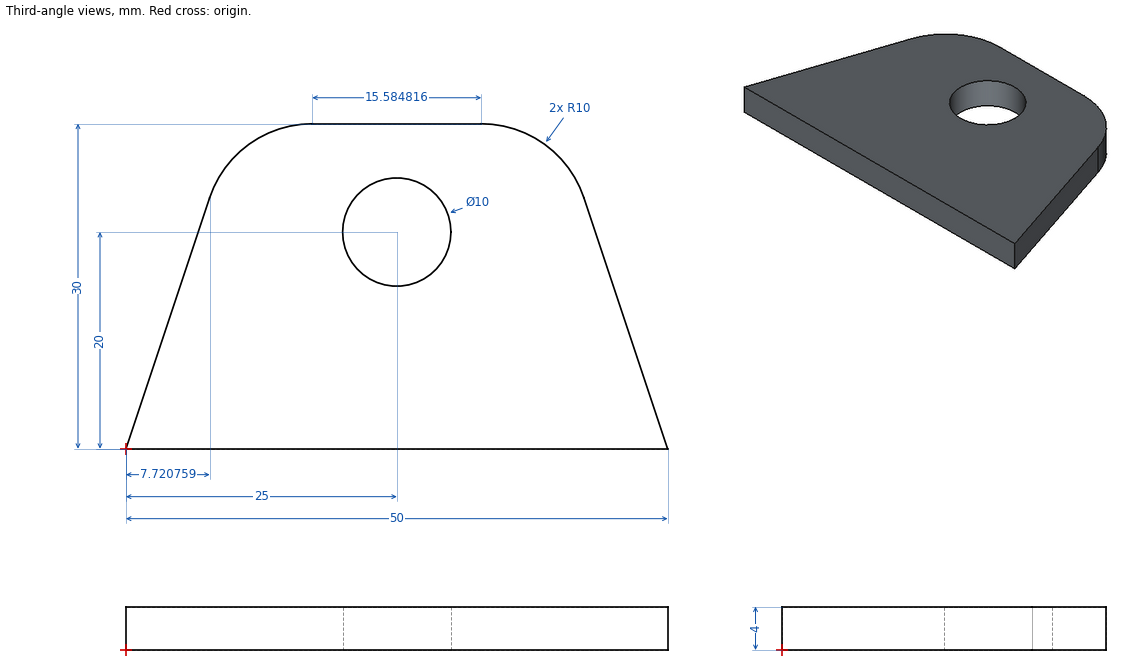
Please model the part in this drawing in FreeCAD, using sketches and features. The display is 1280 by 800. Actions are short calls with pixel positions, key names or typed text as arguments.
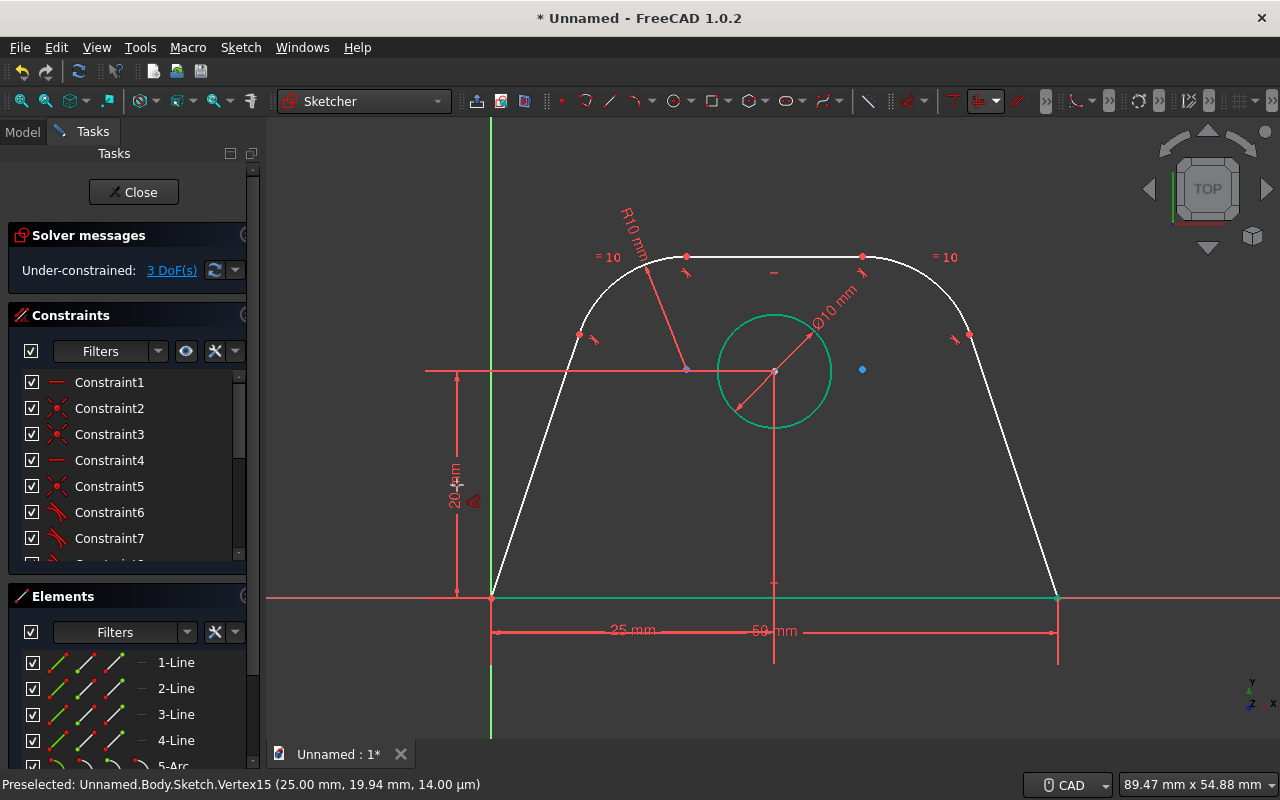
click(862, 257)
click(457, 427)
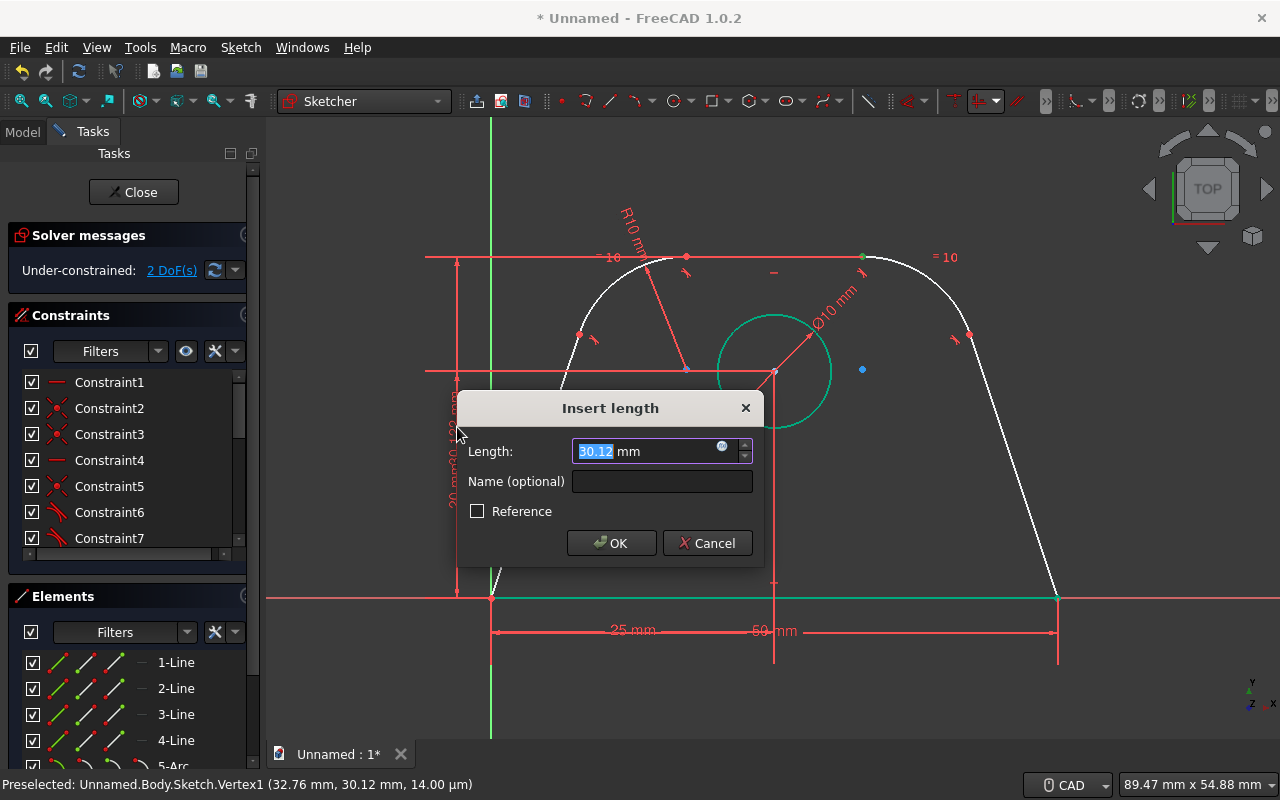
text(30)
key(Return)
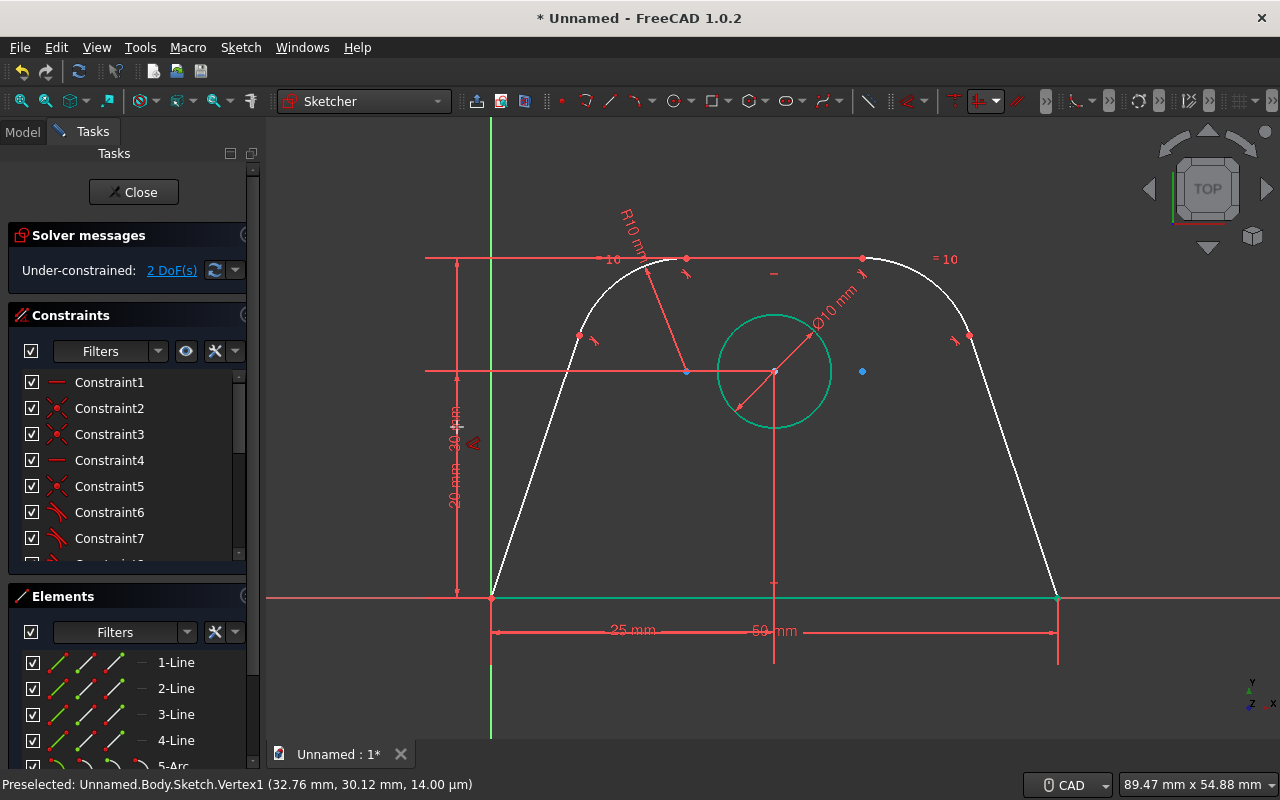
click(810, 258)
click(775, 224)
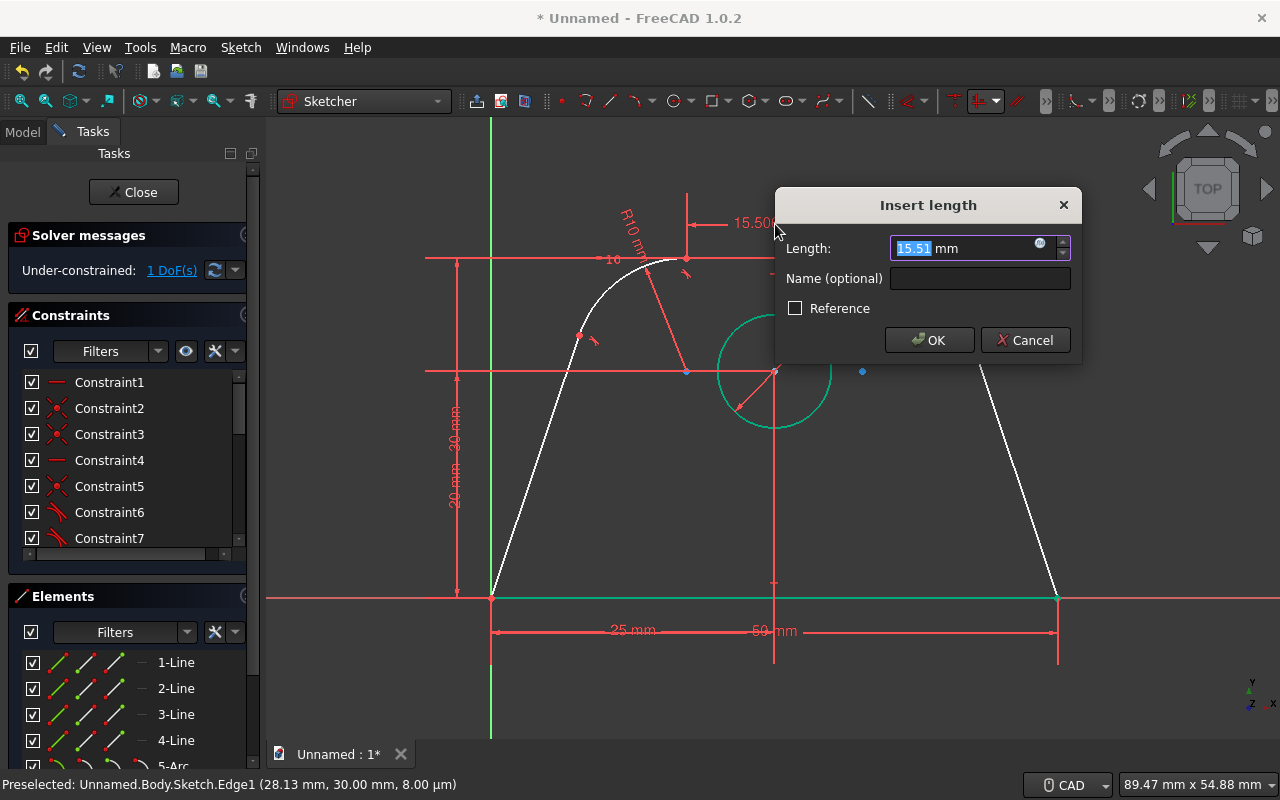
text(15.584816)
key(Return)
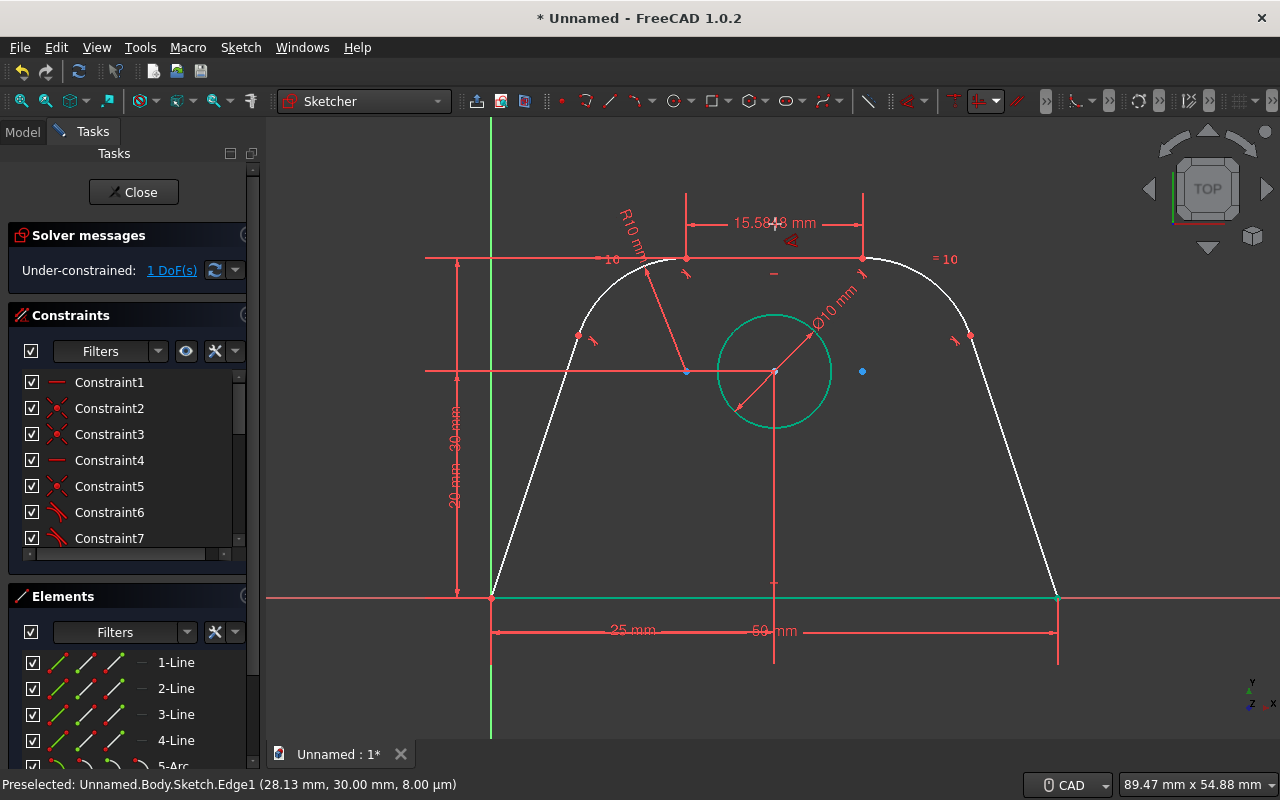
click(579, 336)
click(535, 632)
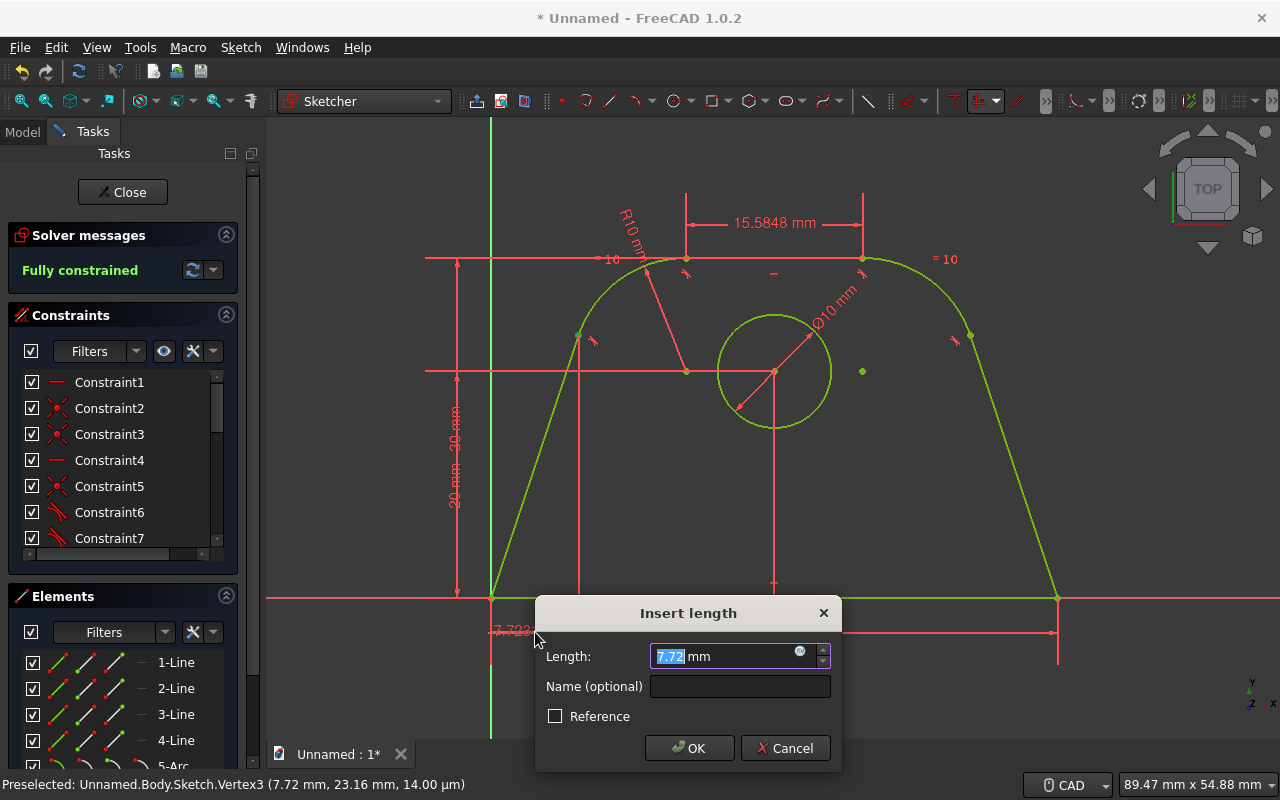
text(7.720759)
key(Return)
key(Escape)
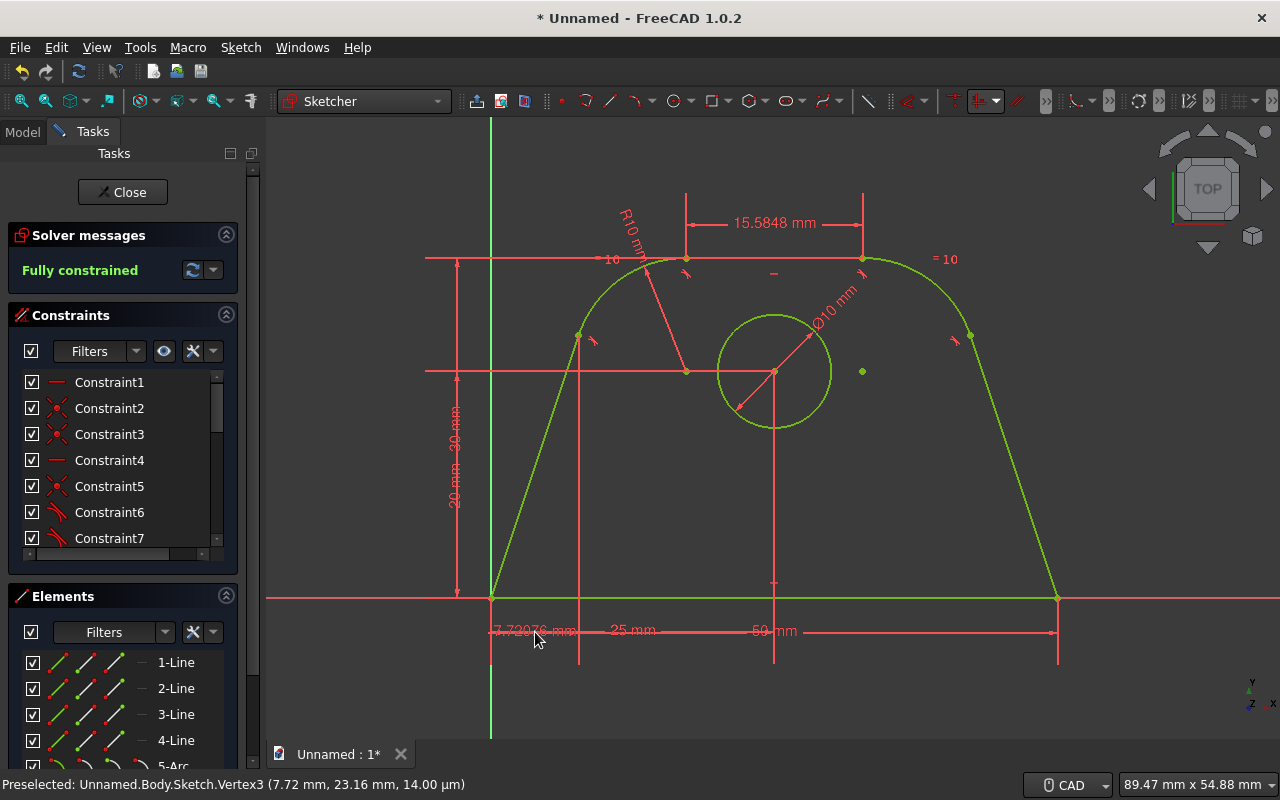
click(123, 192)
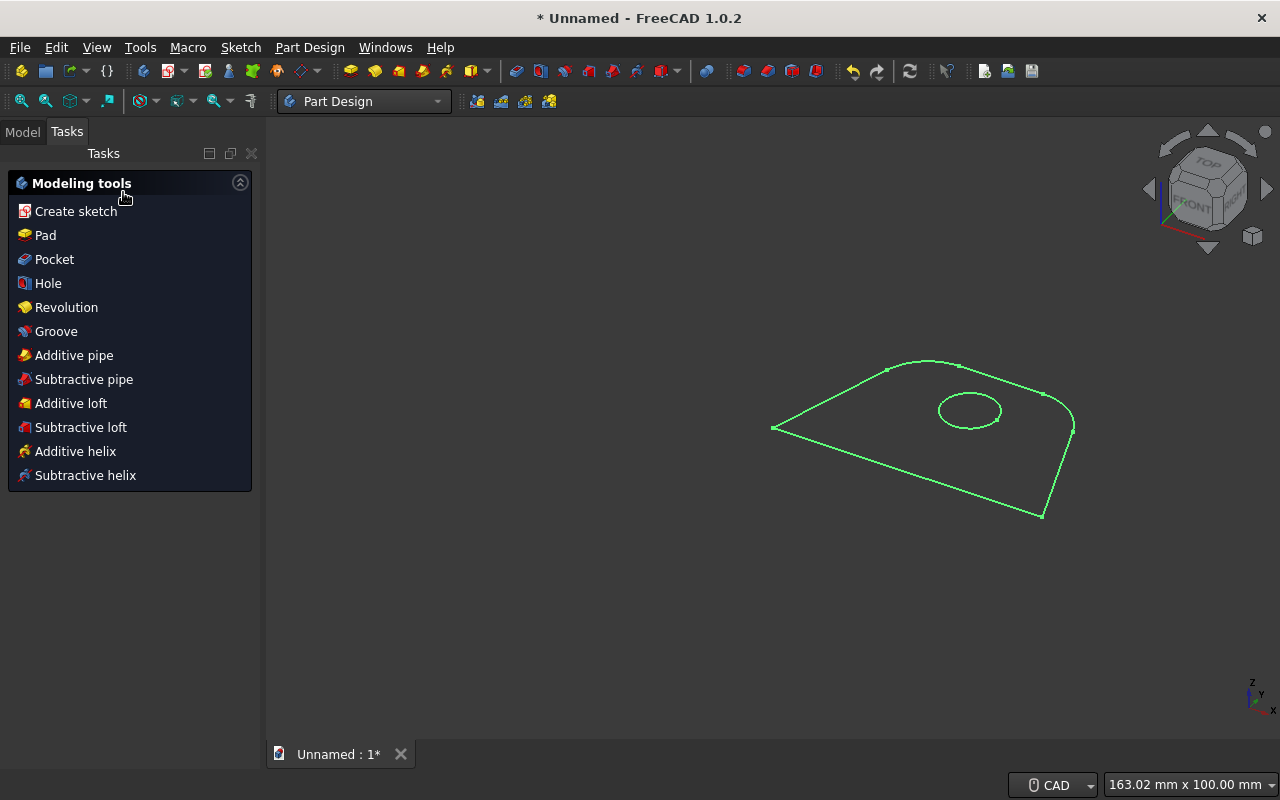
click(352, 72)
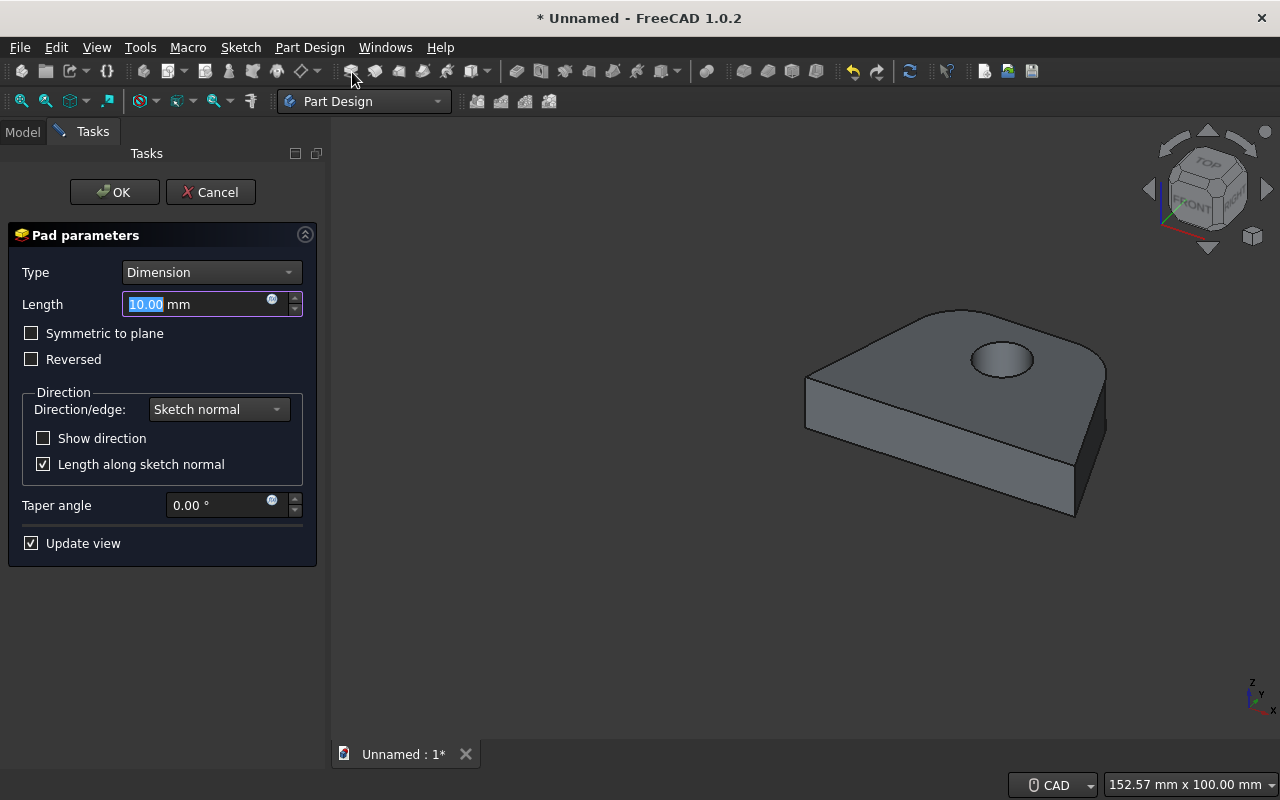
text(4)
key(Tab)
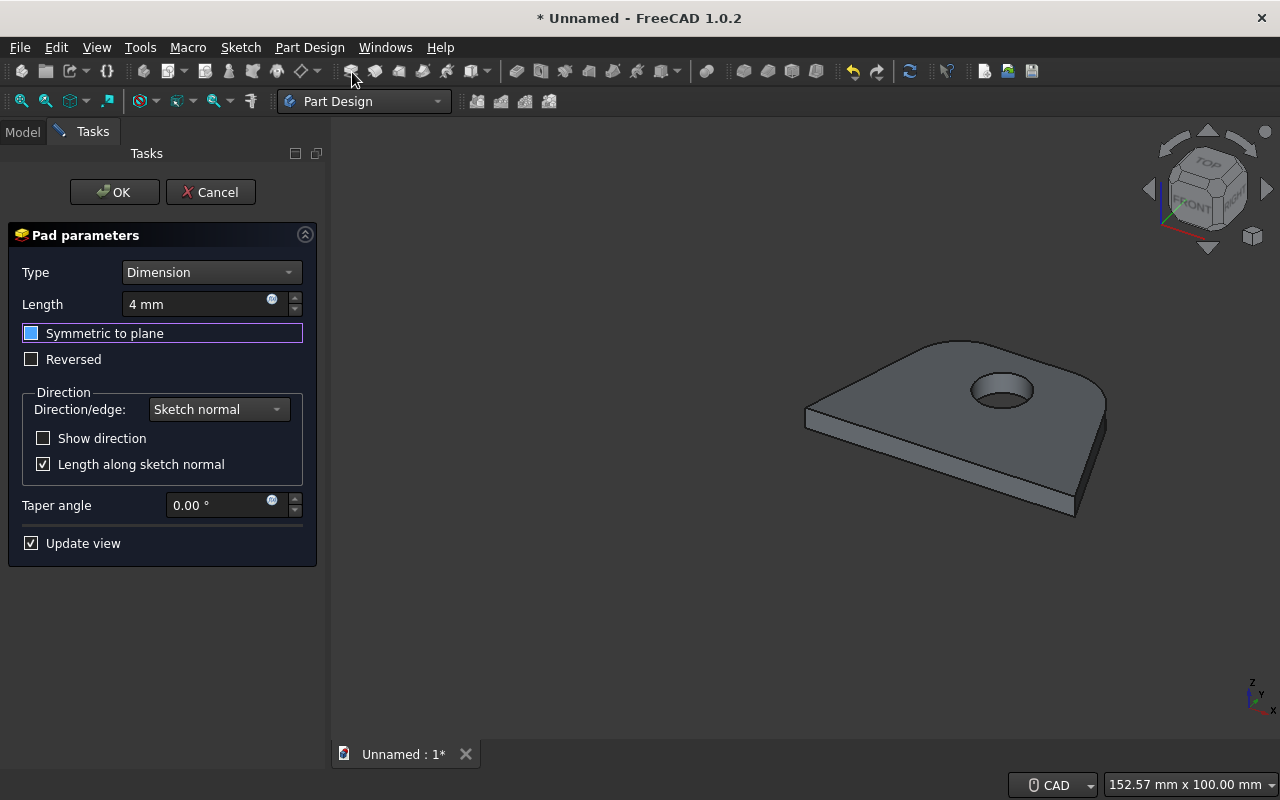
click(115, 192)